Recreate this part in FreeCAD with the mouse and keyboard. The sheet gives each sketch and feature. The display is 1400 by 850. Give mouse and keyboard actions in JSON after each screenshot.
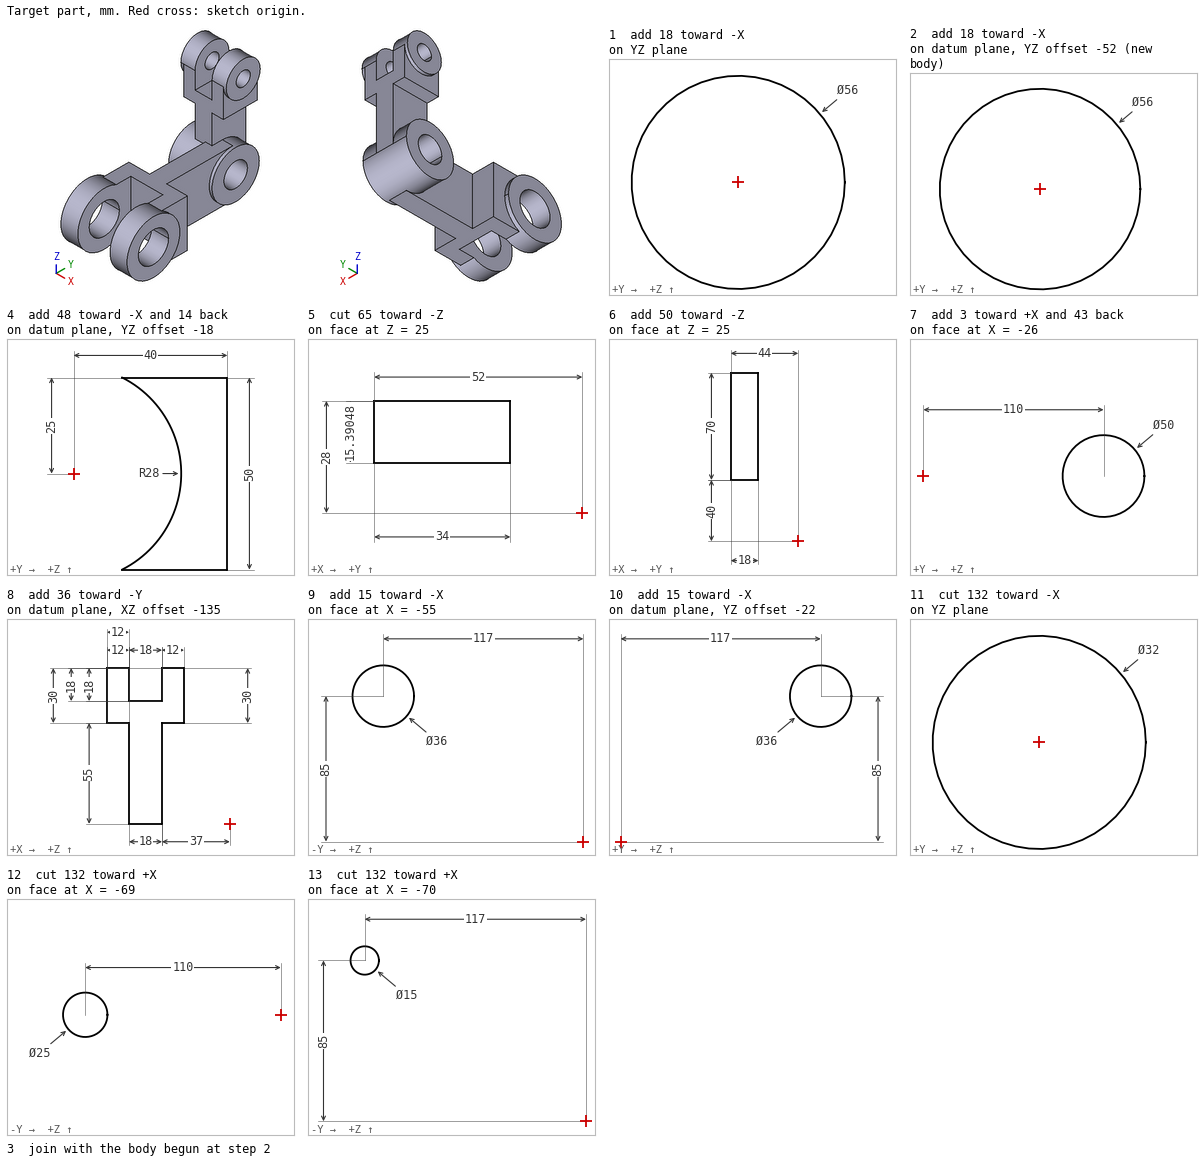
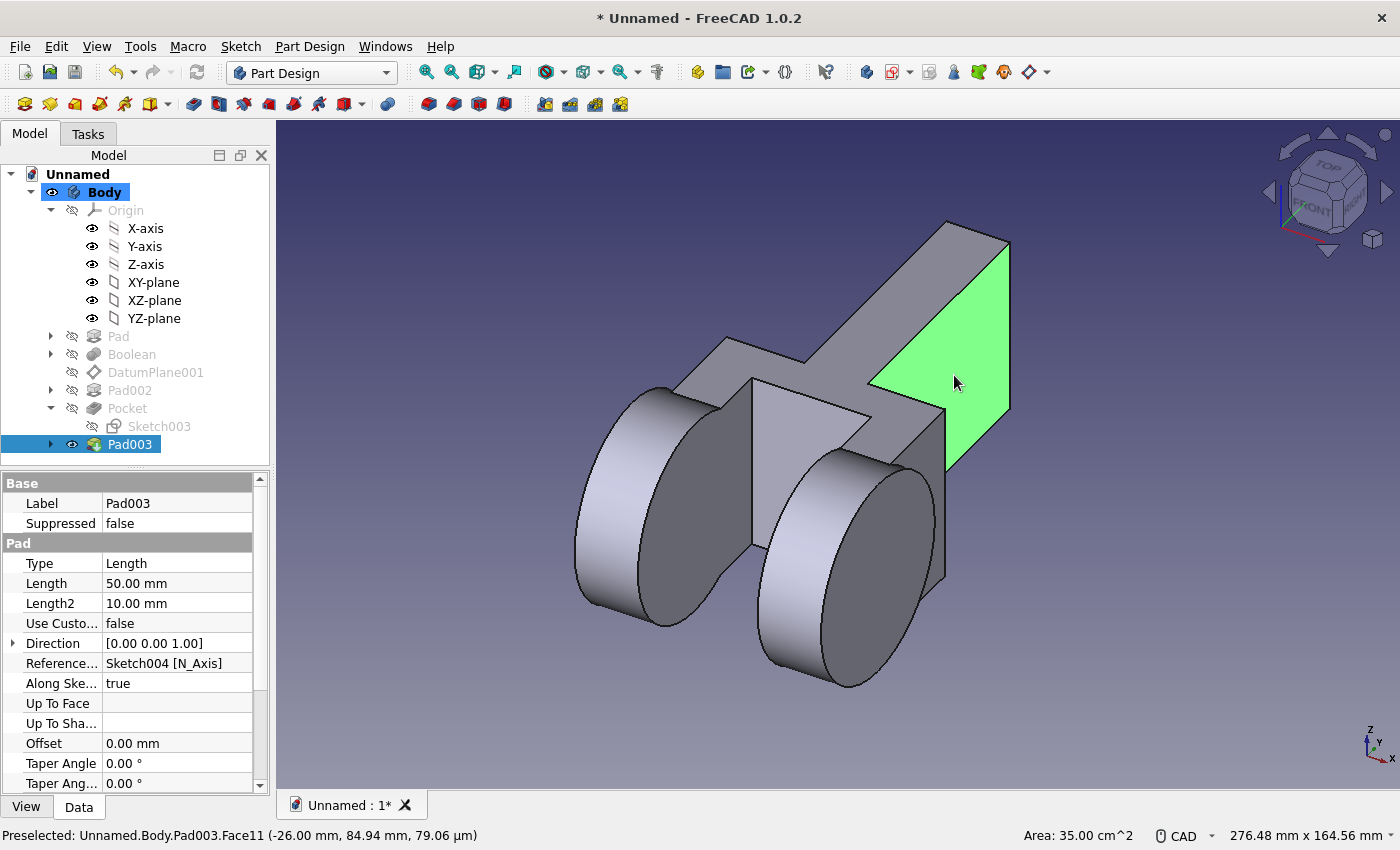
{"action": "left_click", "coordinate": [892, 72]}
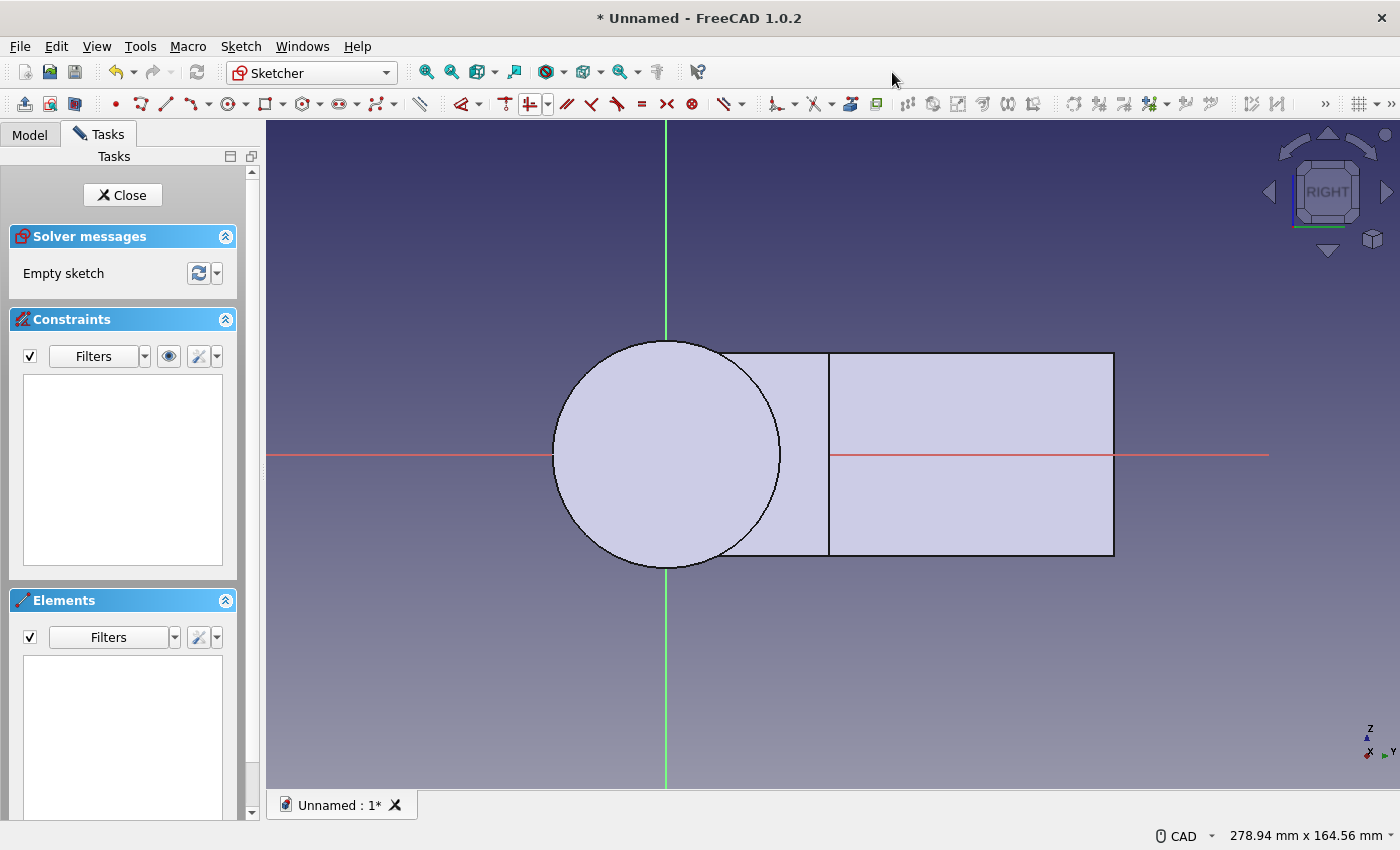
{"action": "key", "text": "q s"}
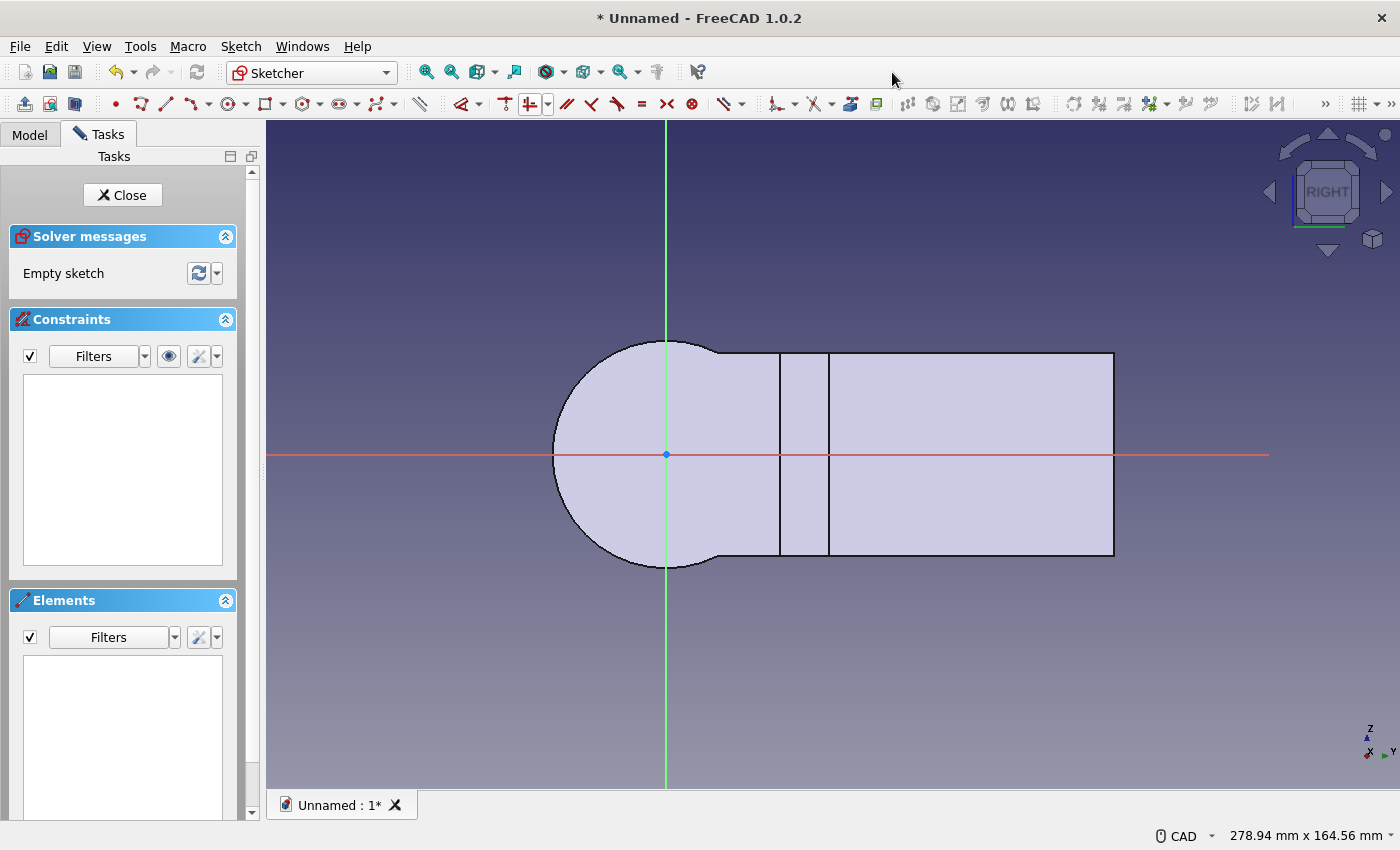
{"action": "scroll", "coordinate": [1235, 455], "scroll_direction": "up", "scroll_amount": 4}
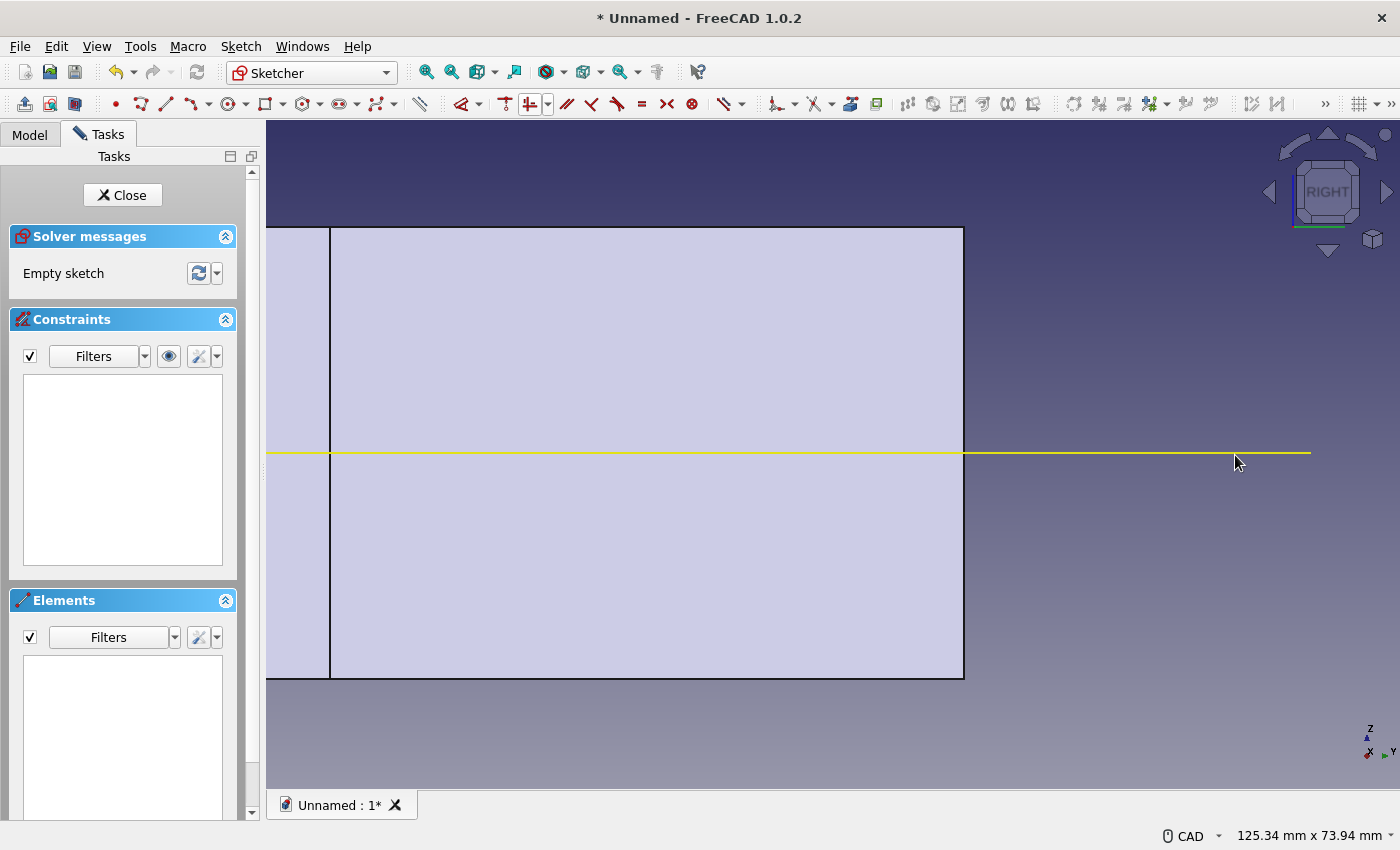
{"action": "key", "text": "g c"}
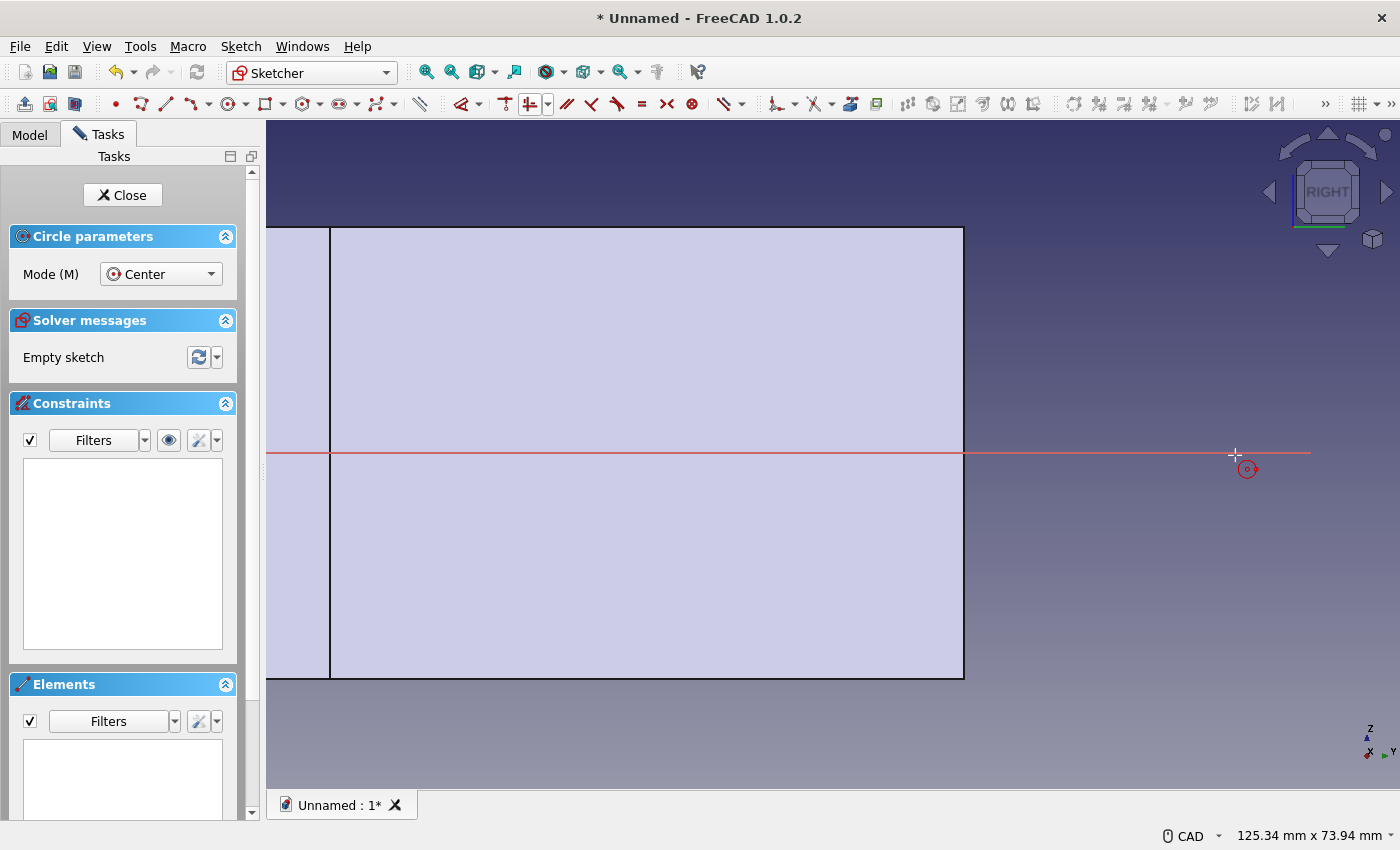
{"action": "left_click", "coordinate": [964, 453]}
{"action": "left_click", "coordinate": [1124, 293]}
{"action": "key", "text": "Escape"}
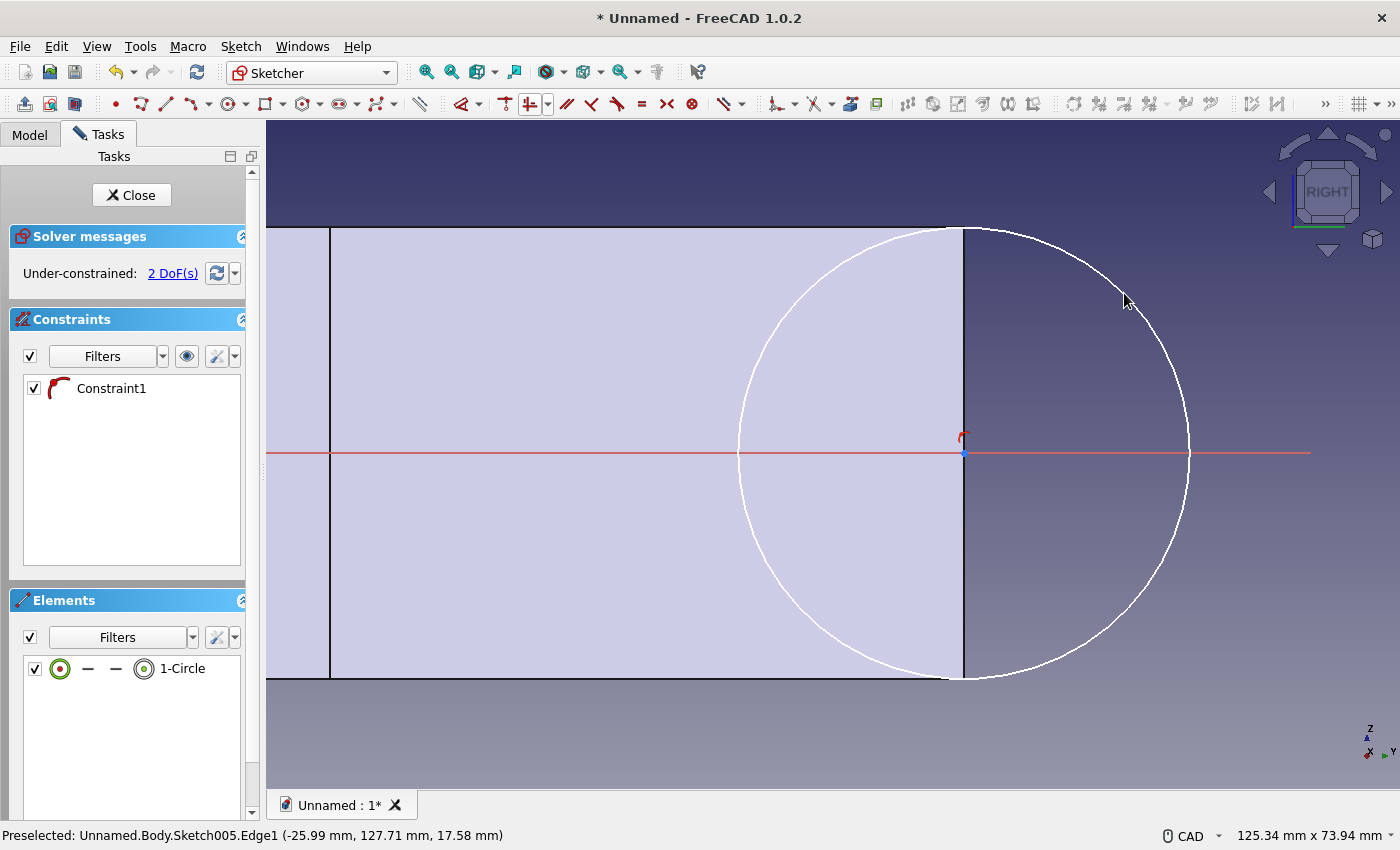
{"action": "left_click", "coordinate": [1123, 293]}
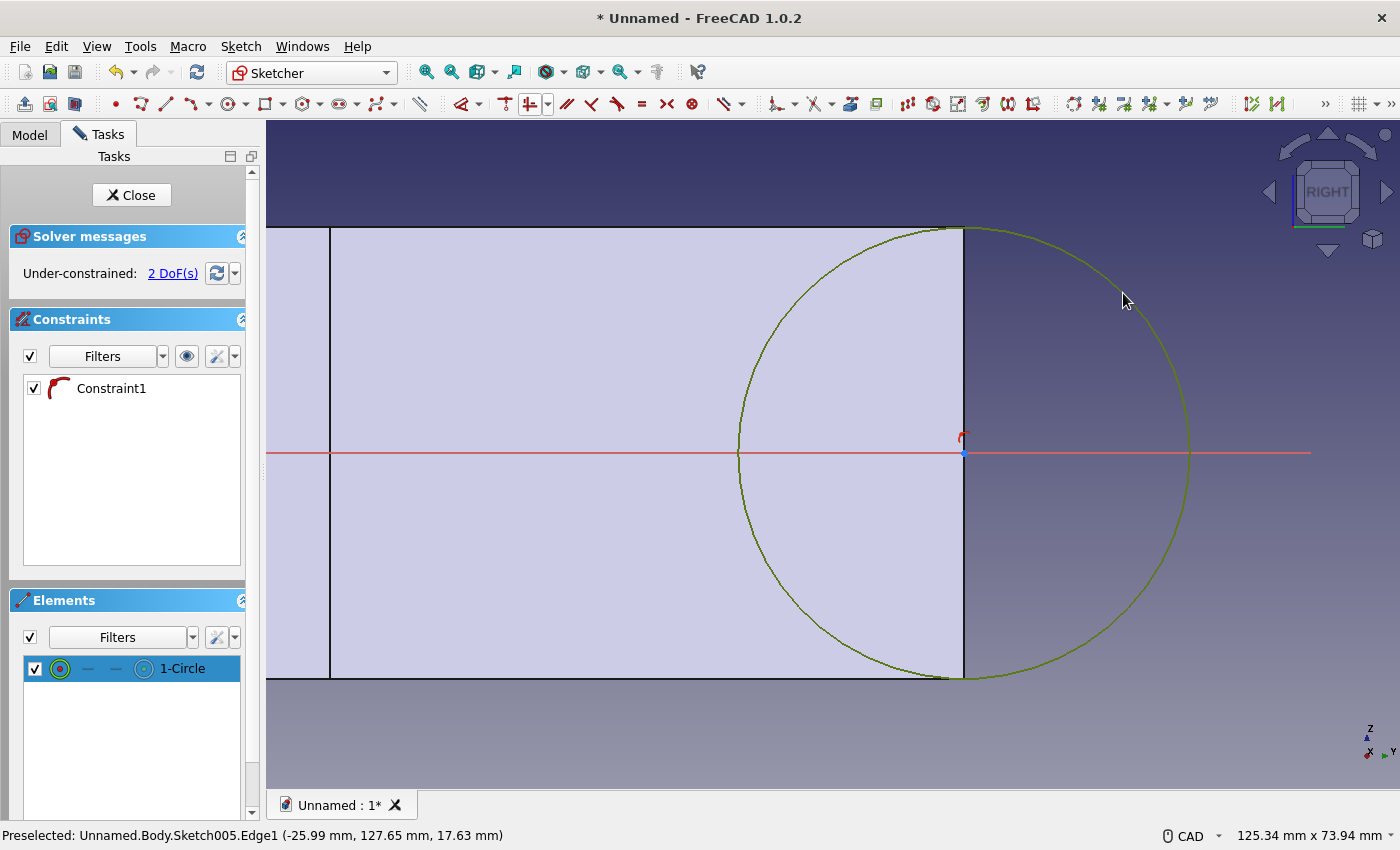
{"action": "key", "text": "k o"}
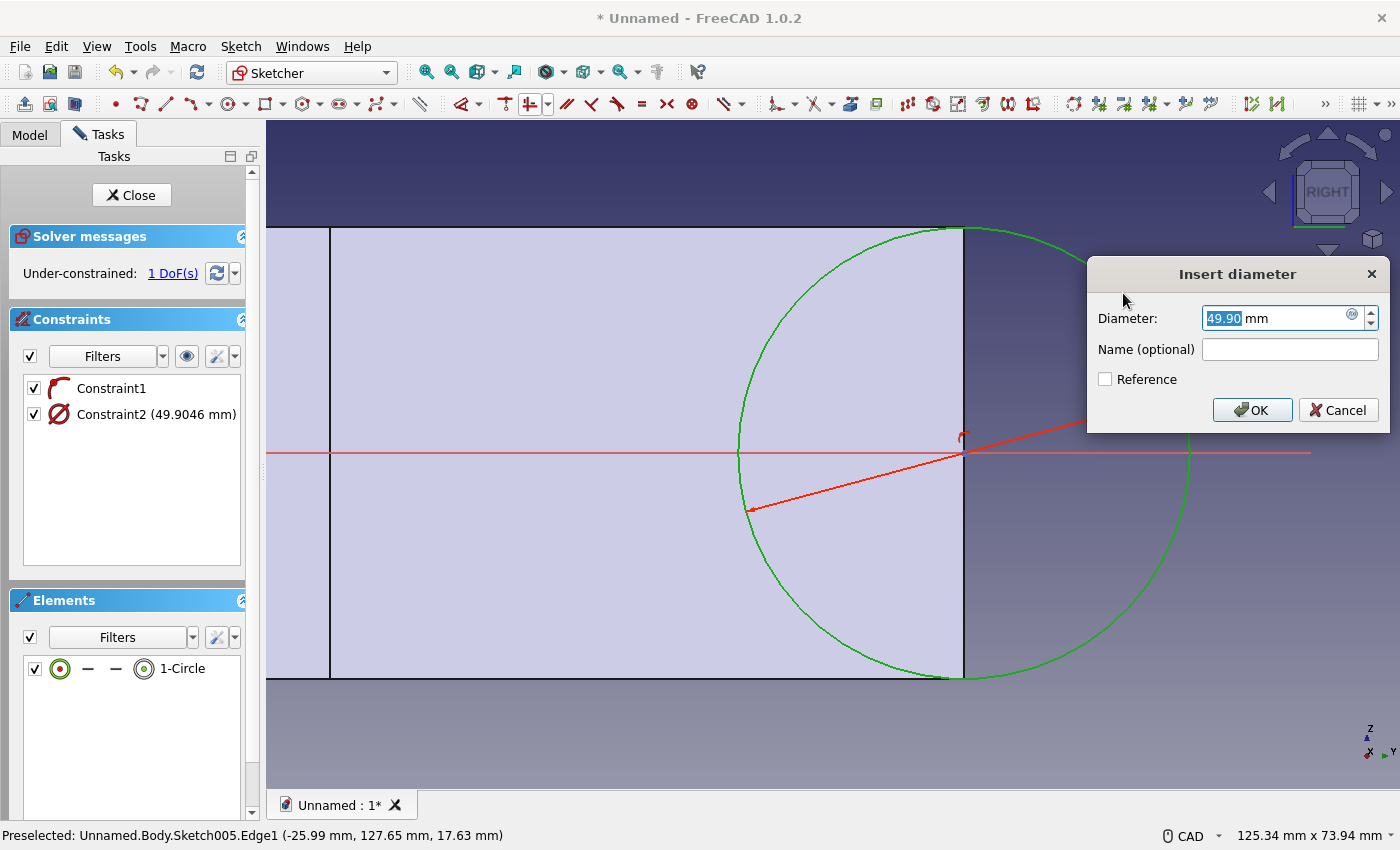
{"action": "type", "text": "50"}
{"action": "key", "text": "Return"}